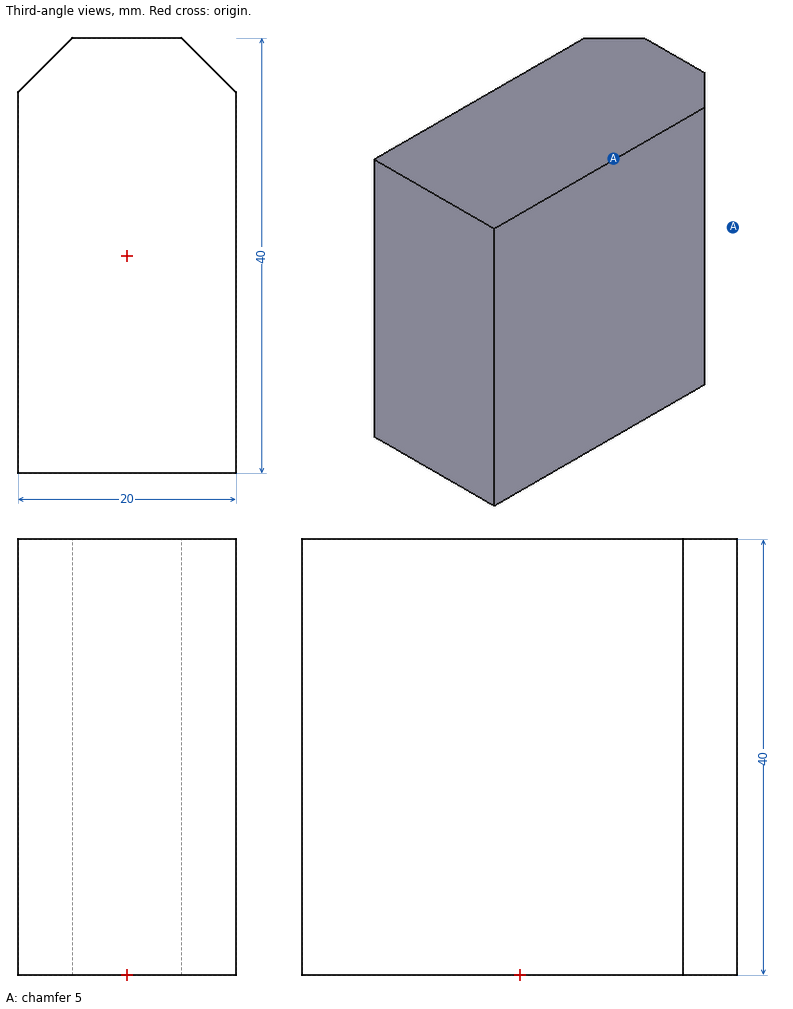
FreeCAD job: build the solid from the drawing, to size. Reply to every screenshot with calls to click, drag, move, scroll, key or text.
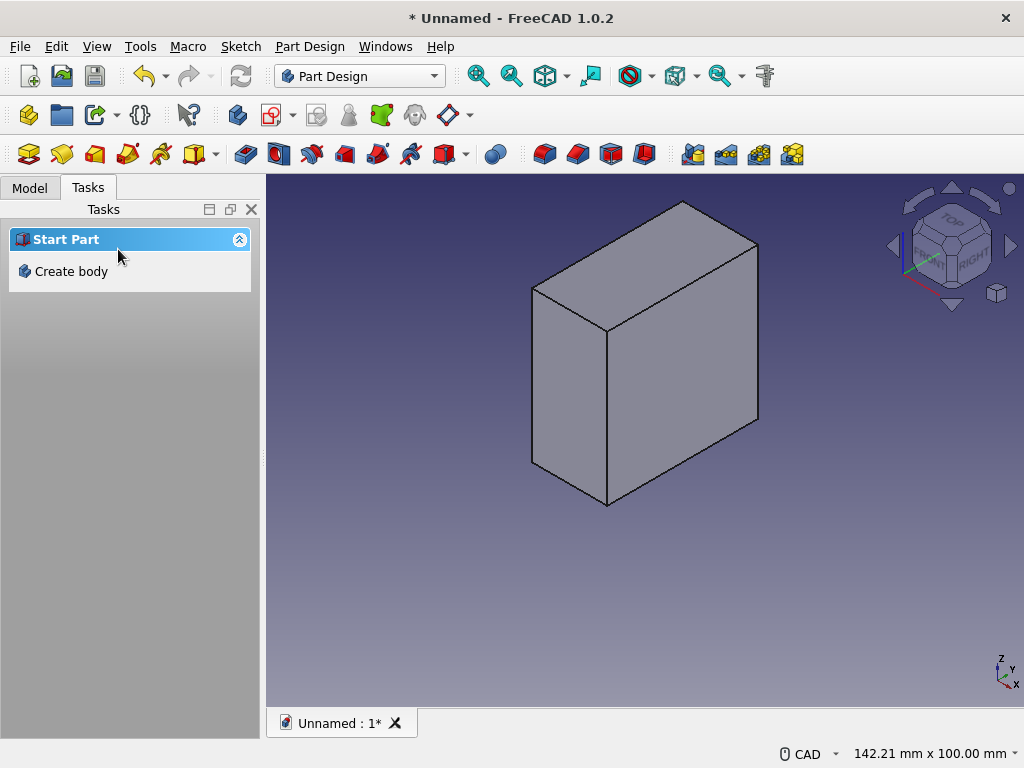
key(2)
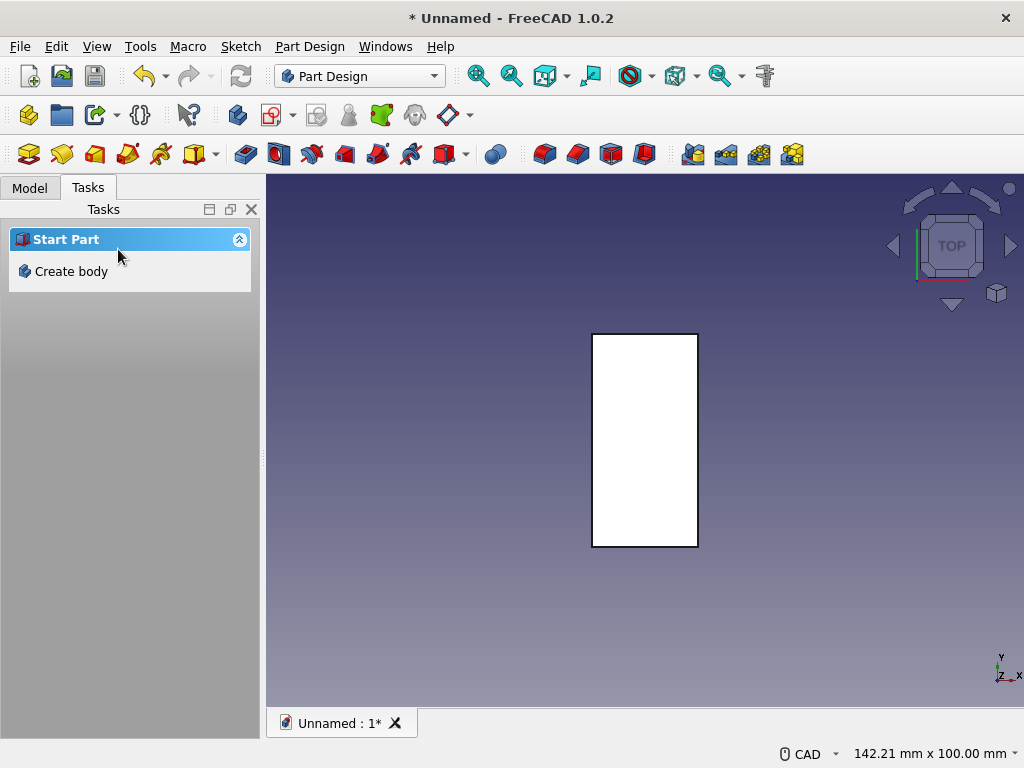
click(479, 76)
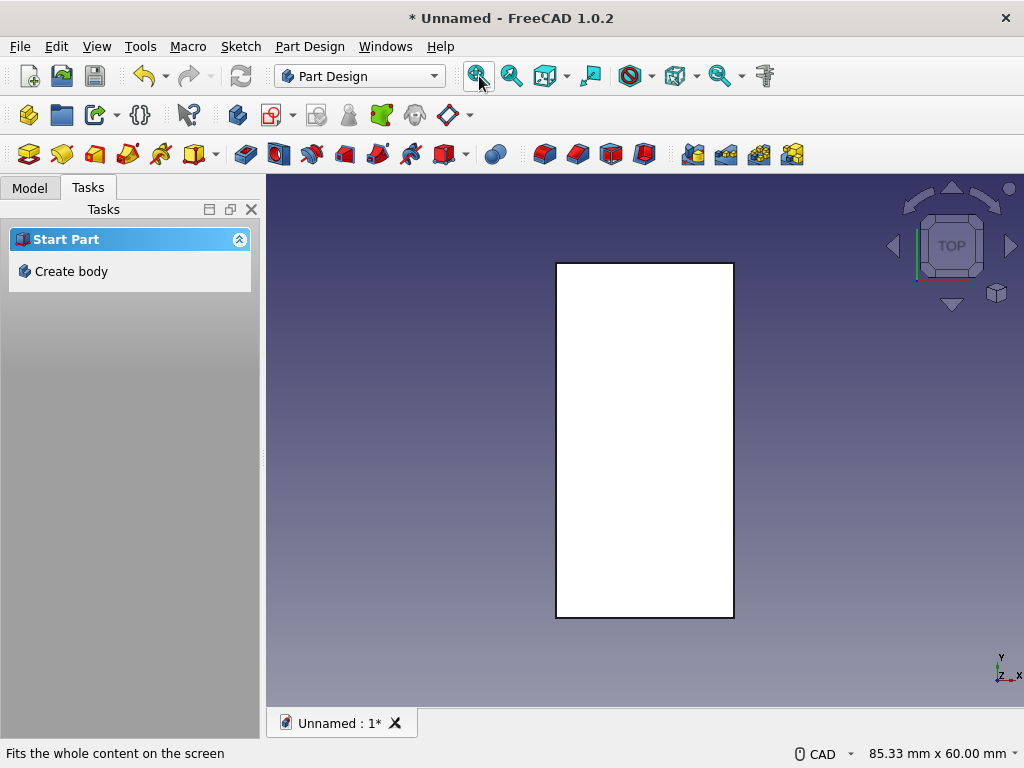
key(1)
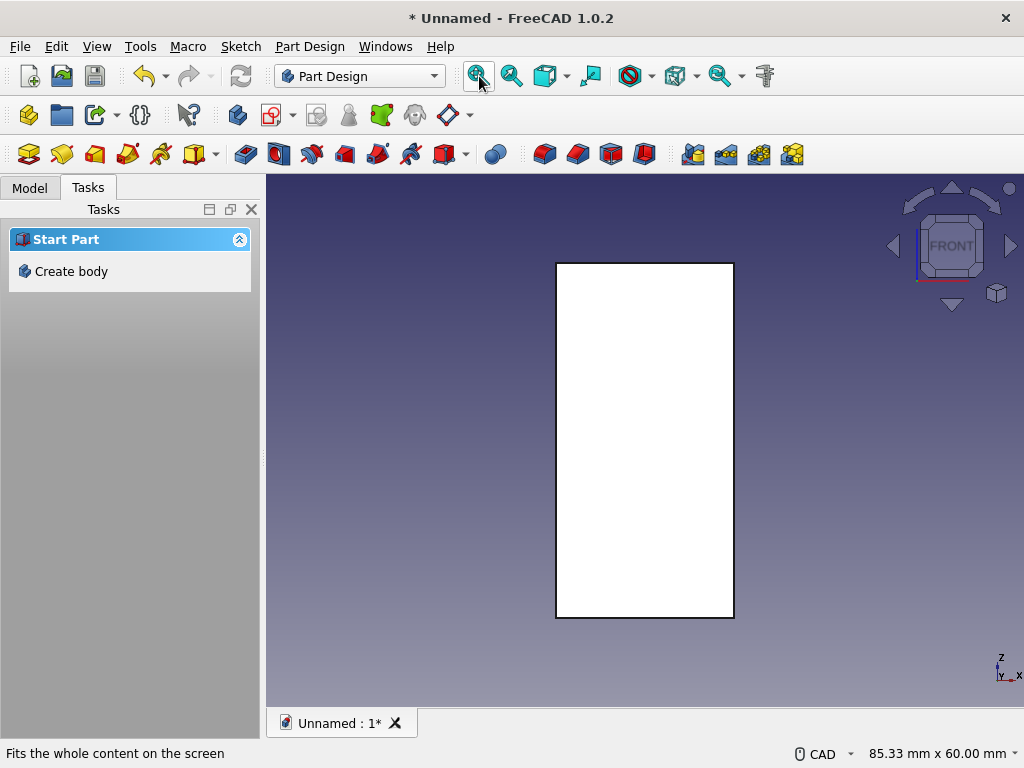
key(3)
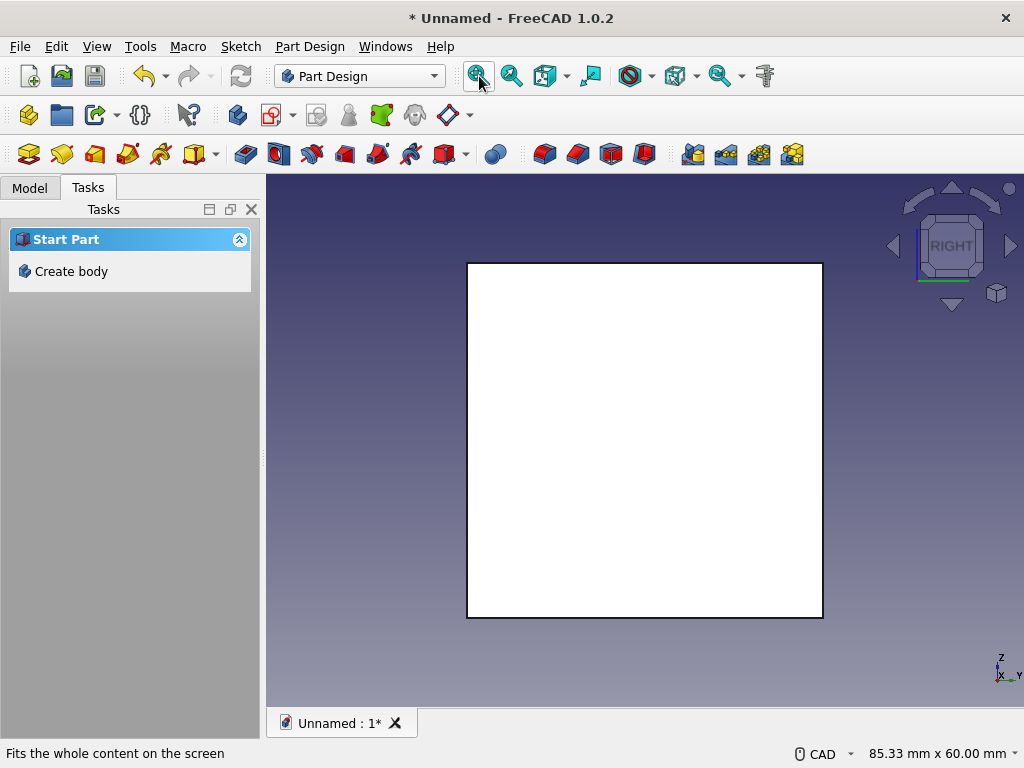
click(823, 439)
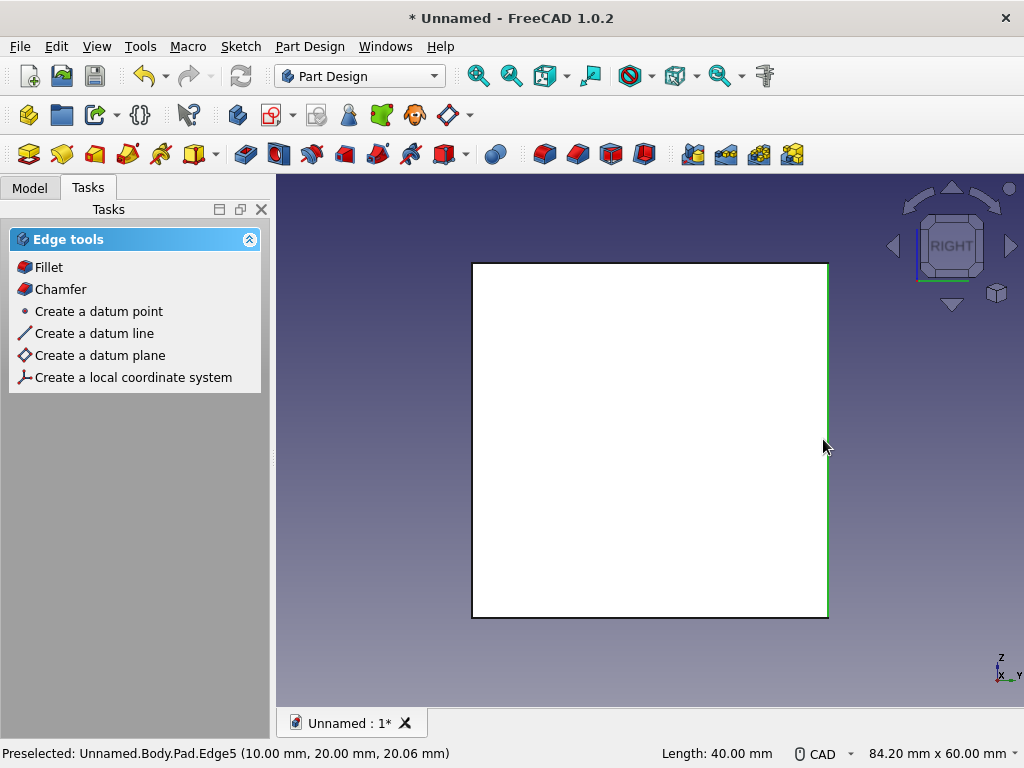
key(5)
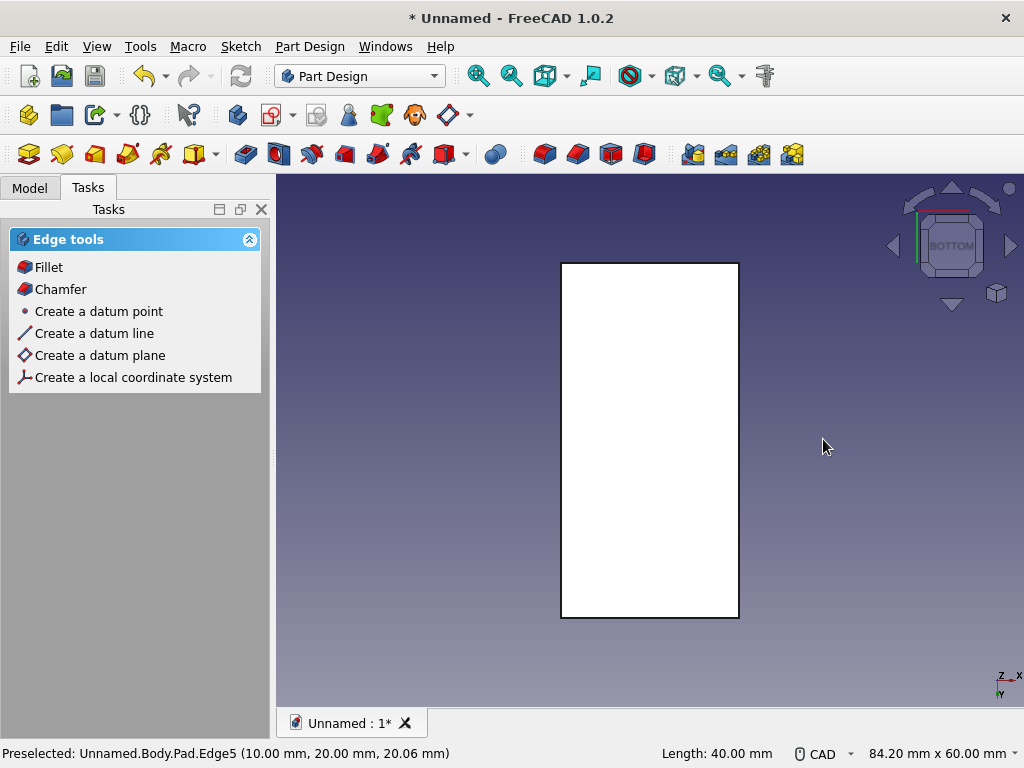
key(4)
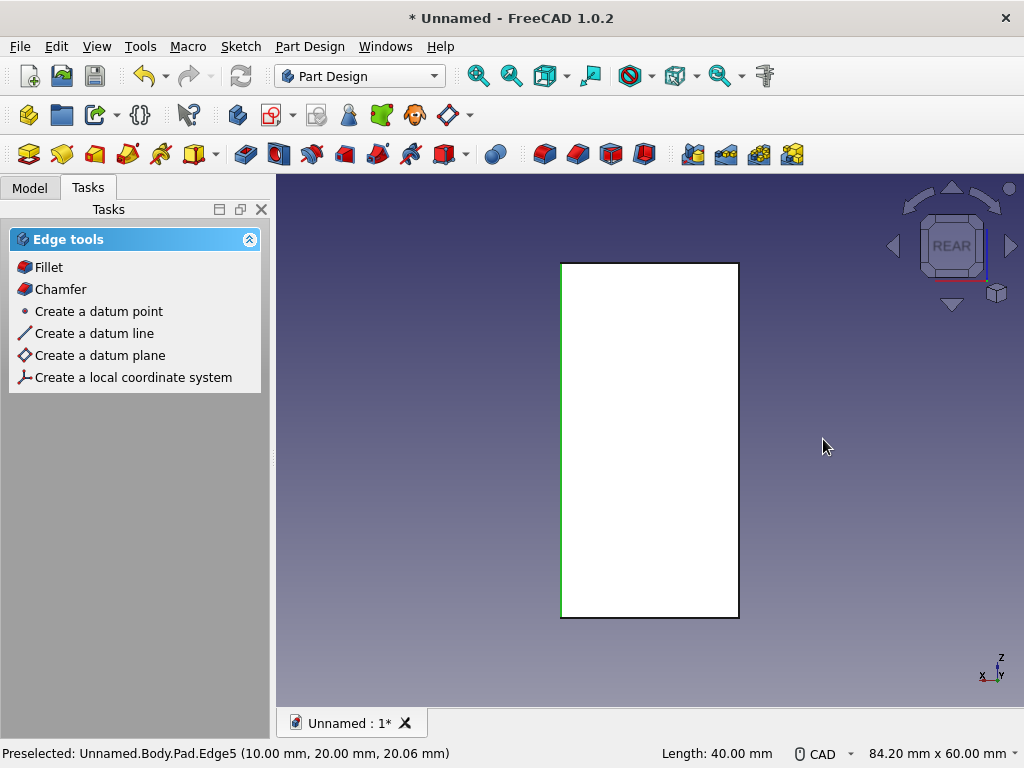
click(739, 439, ctrl)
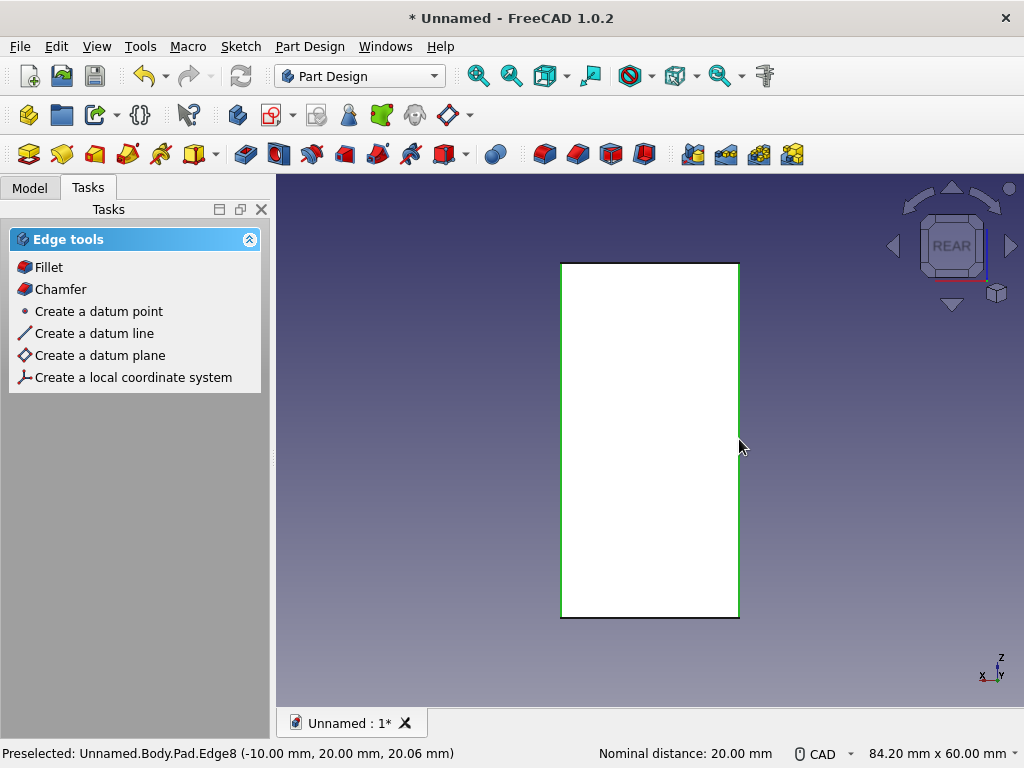
click(578, 154)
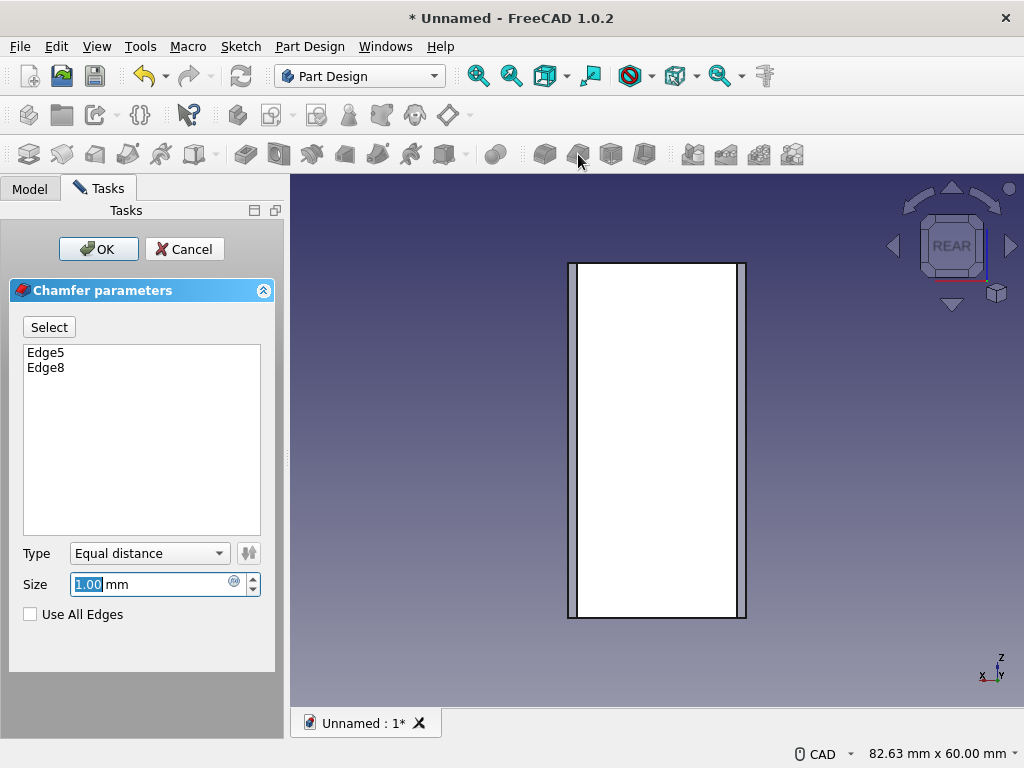
text(5)
key(Tab)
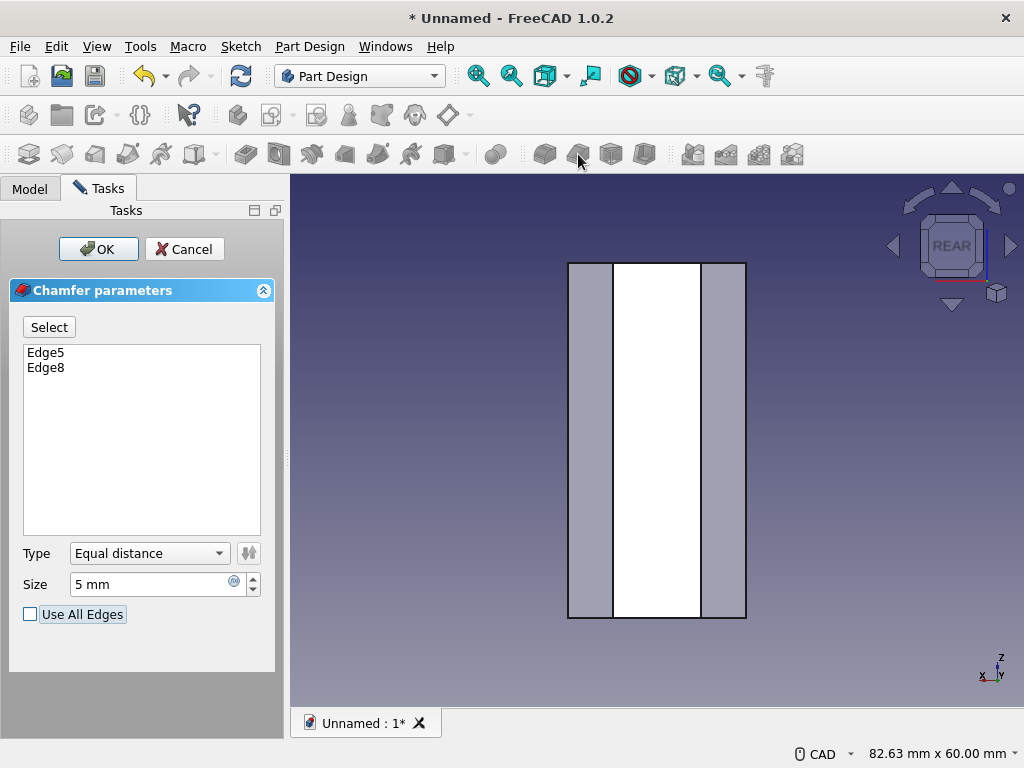
click(99, 249)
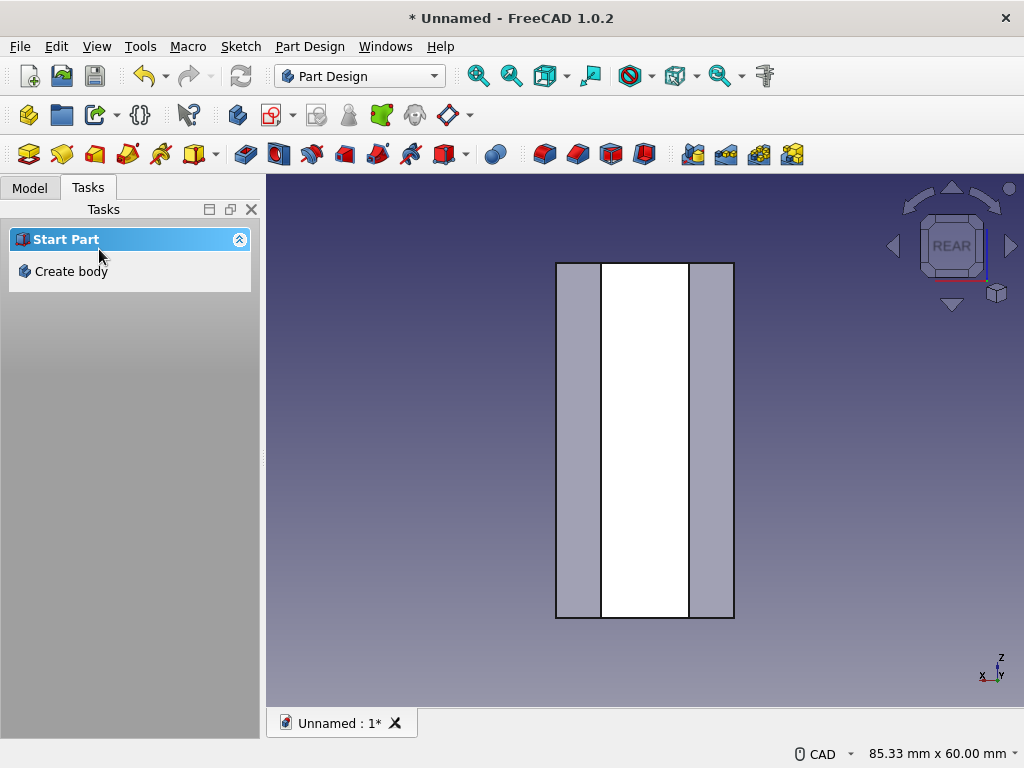
key(0)